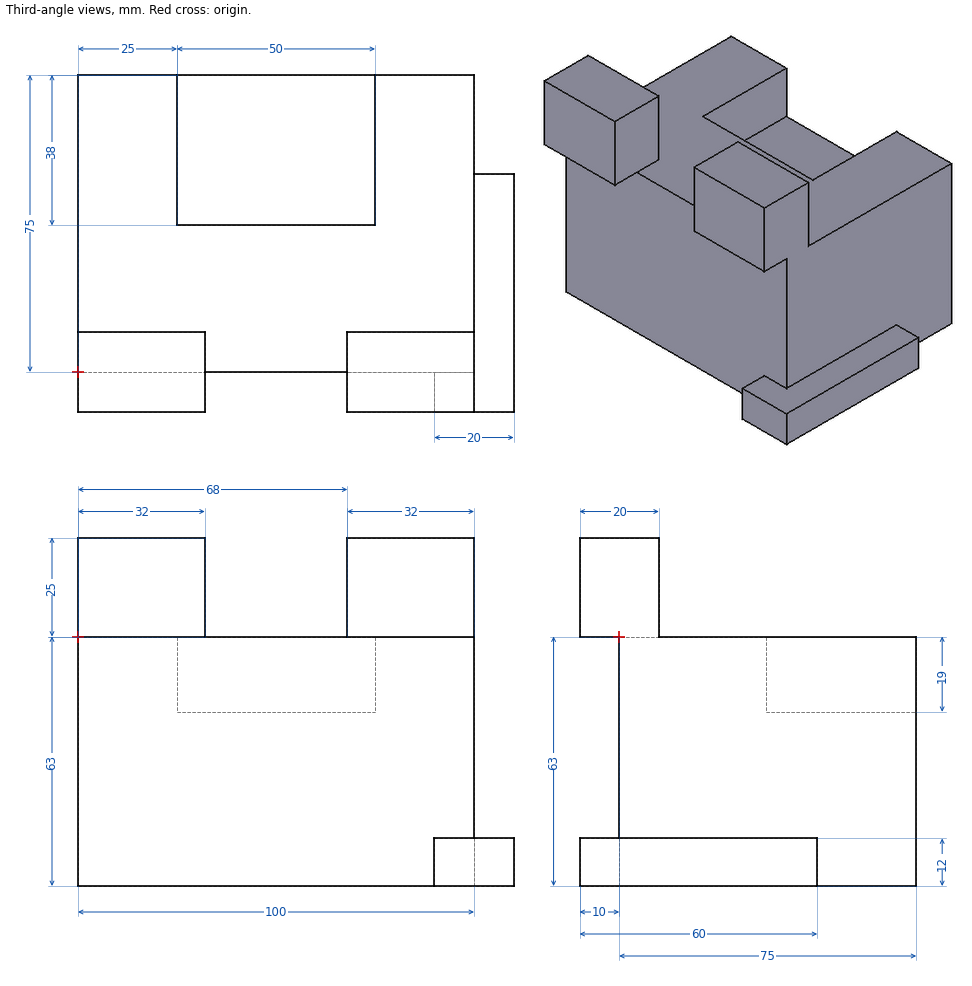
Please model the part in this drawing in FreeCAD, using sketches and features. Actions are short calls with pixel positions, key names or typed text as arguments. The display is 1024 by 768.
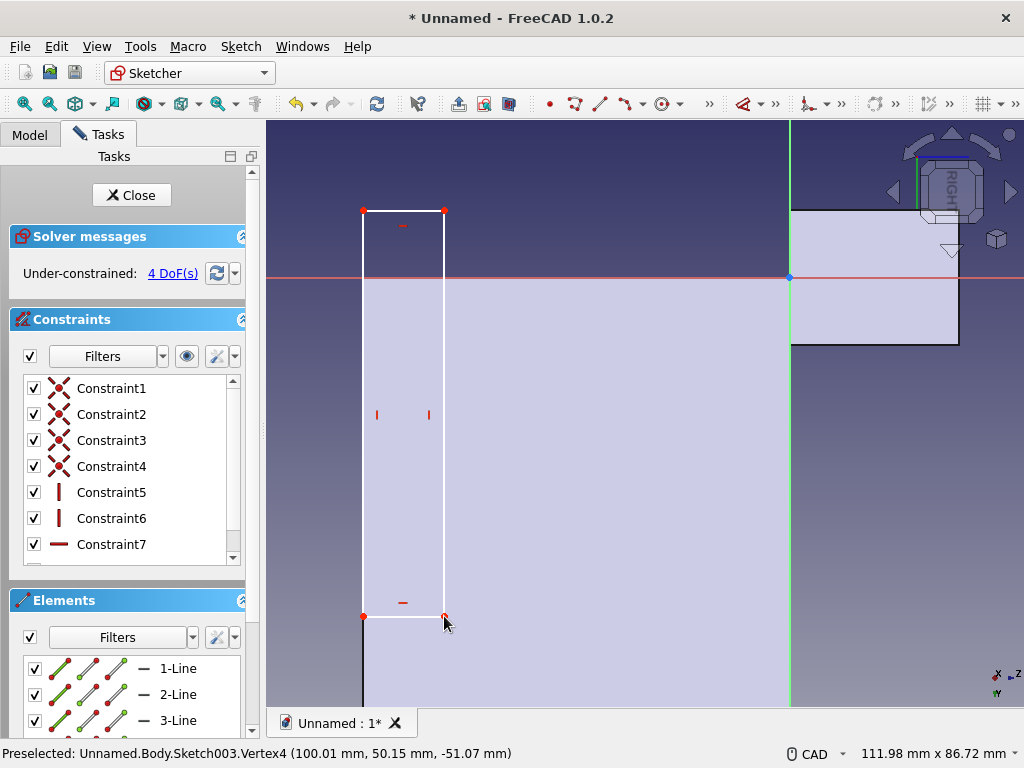
click(742, 104)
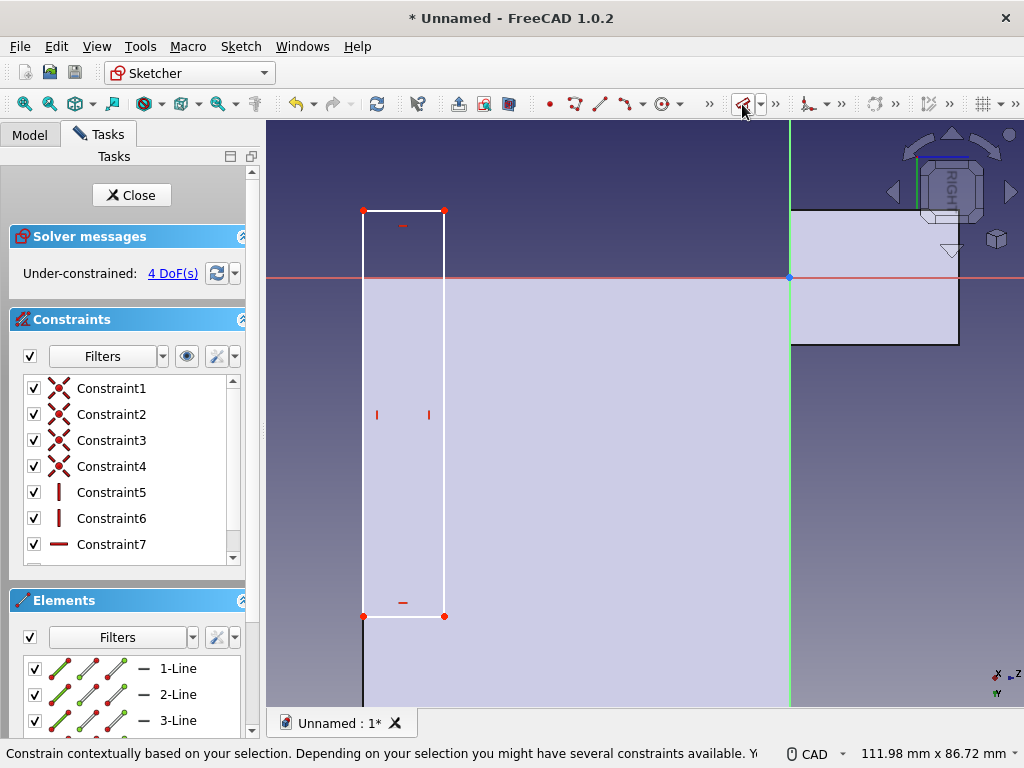
click(363, 333)
click(329, 414)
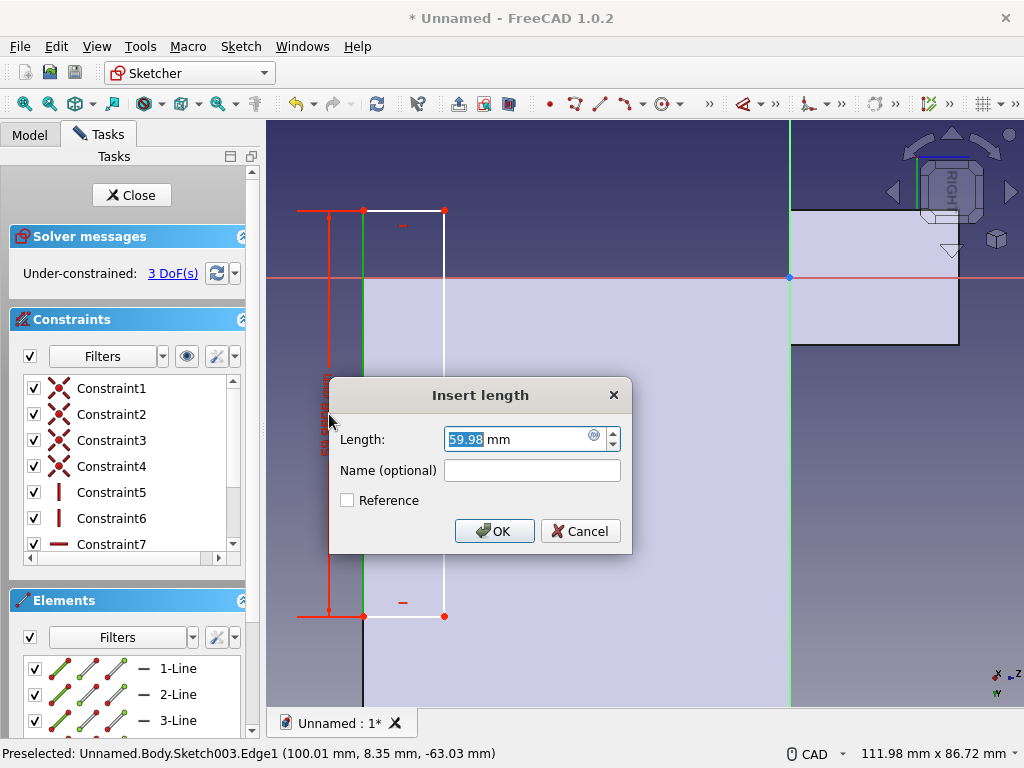
text(60)
key(Return)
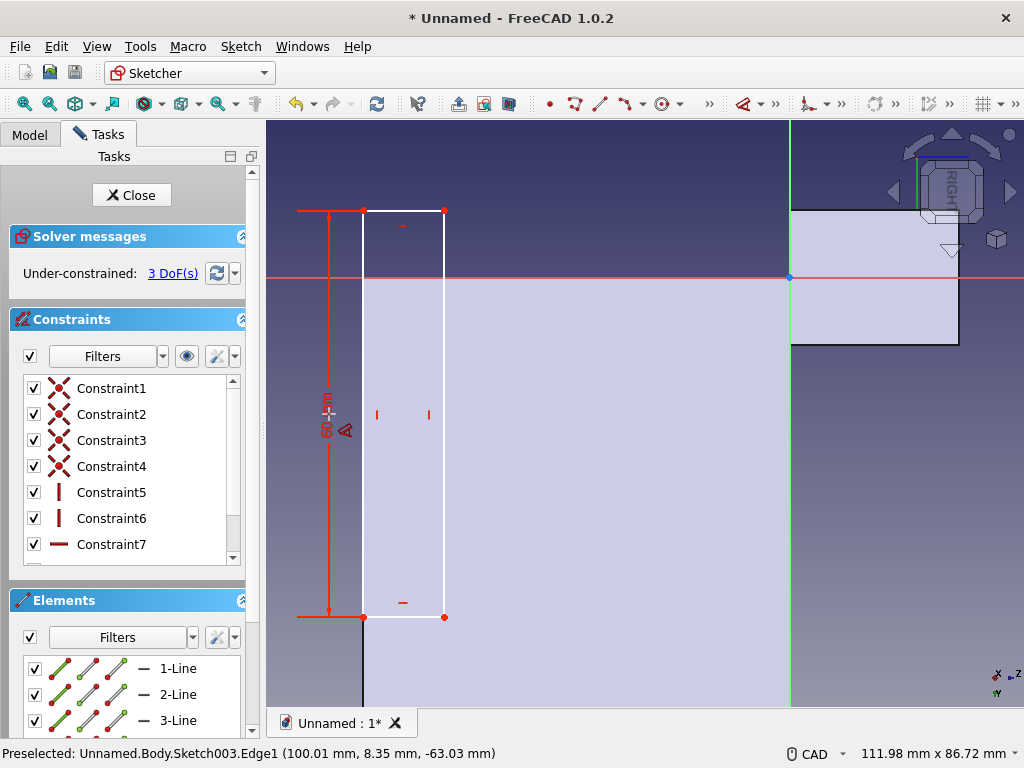
click(387, 617)
click(404, 651)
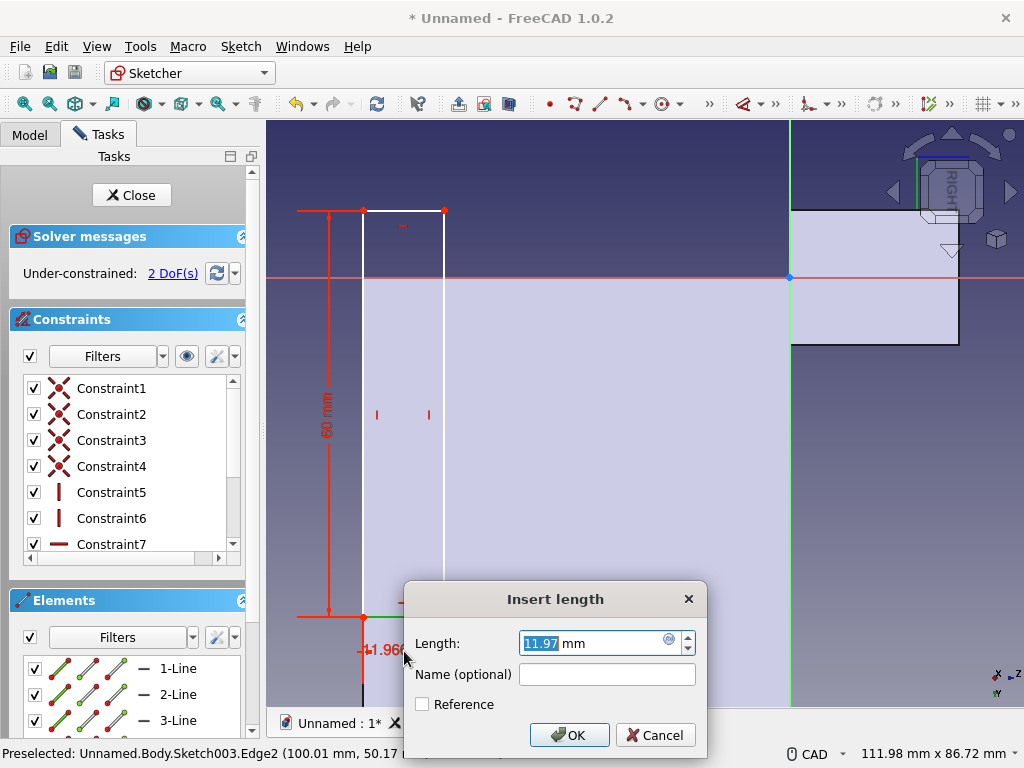
text(12)
key(Return)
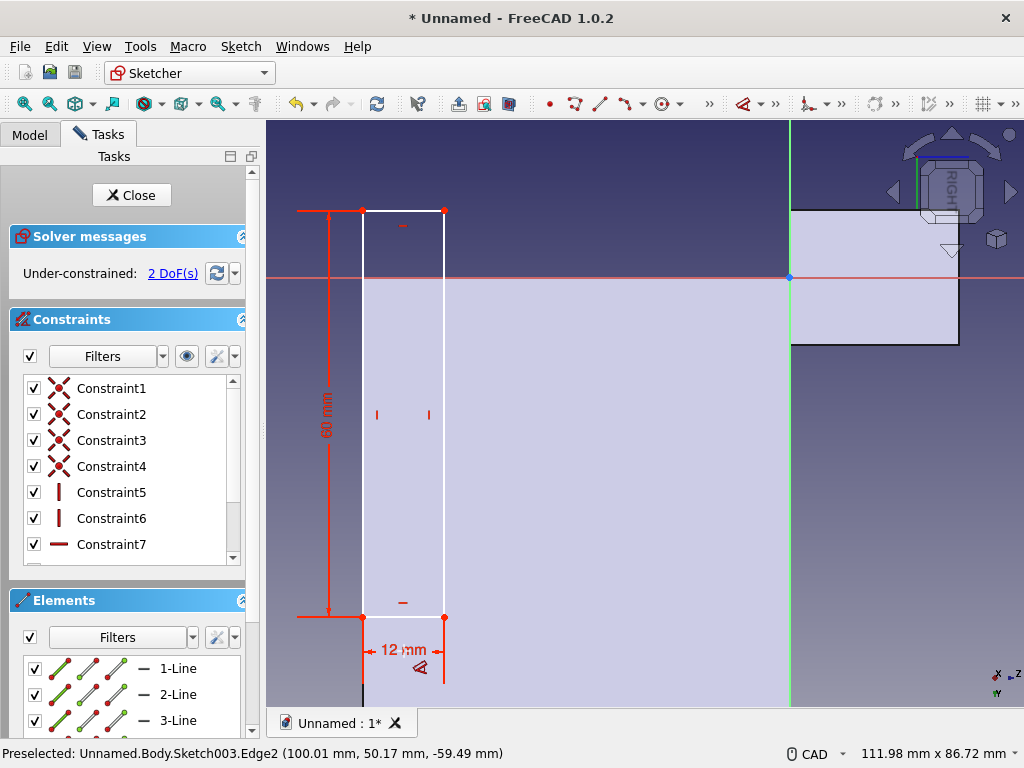
click(363, 211)
click(576, 177)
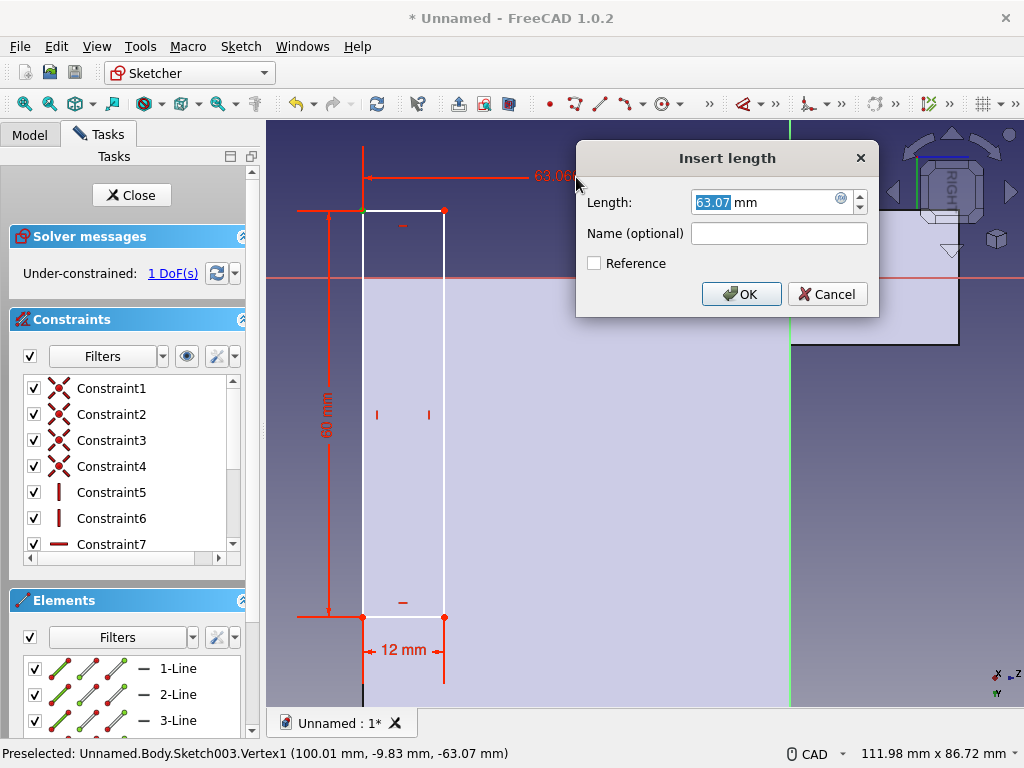
text(63)
key(Return)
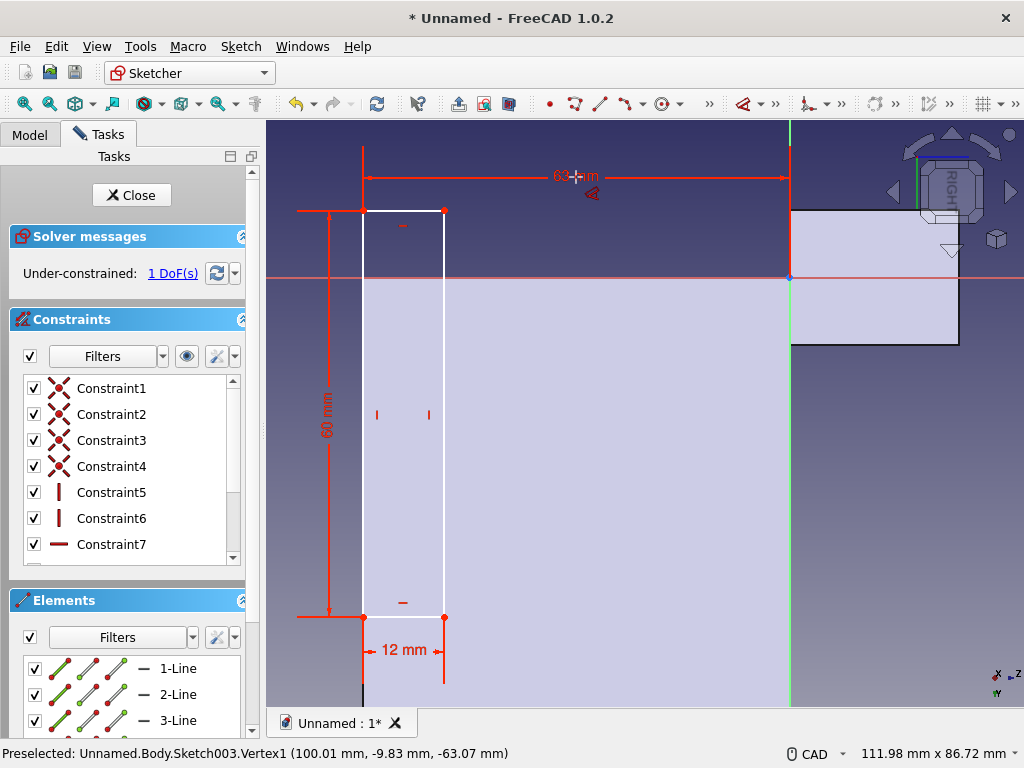
click(363, 211)
click(824, 244)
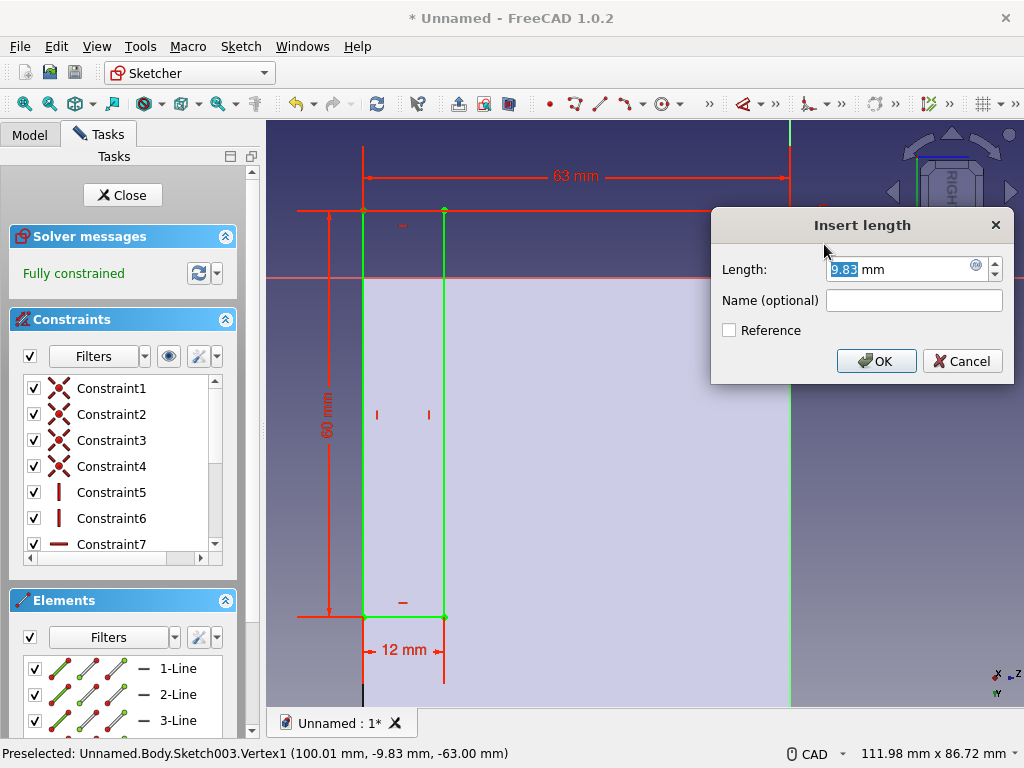
text(10)
key(Return)
key(Escape)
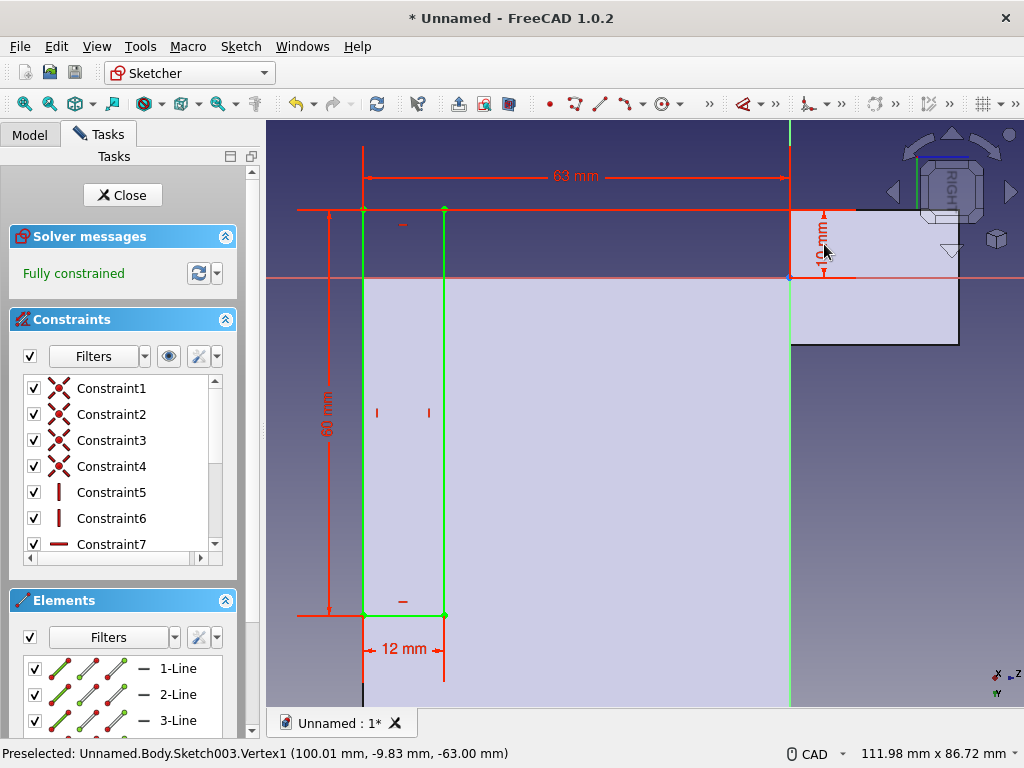
click(123, 195)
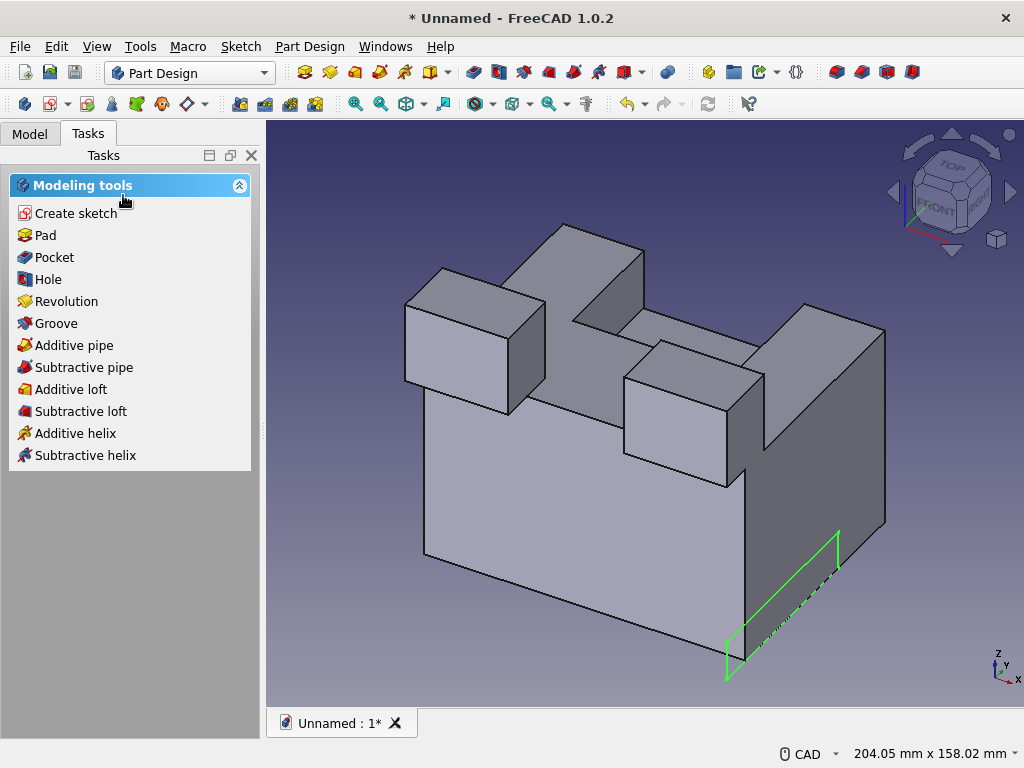
click(305, 72)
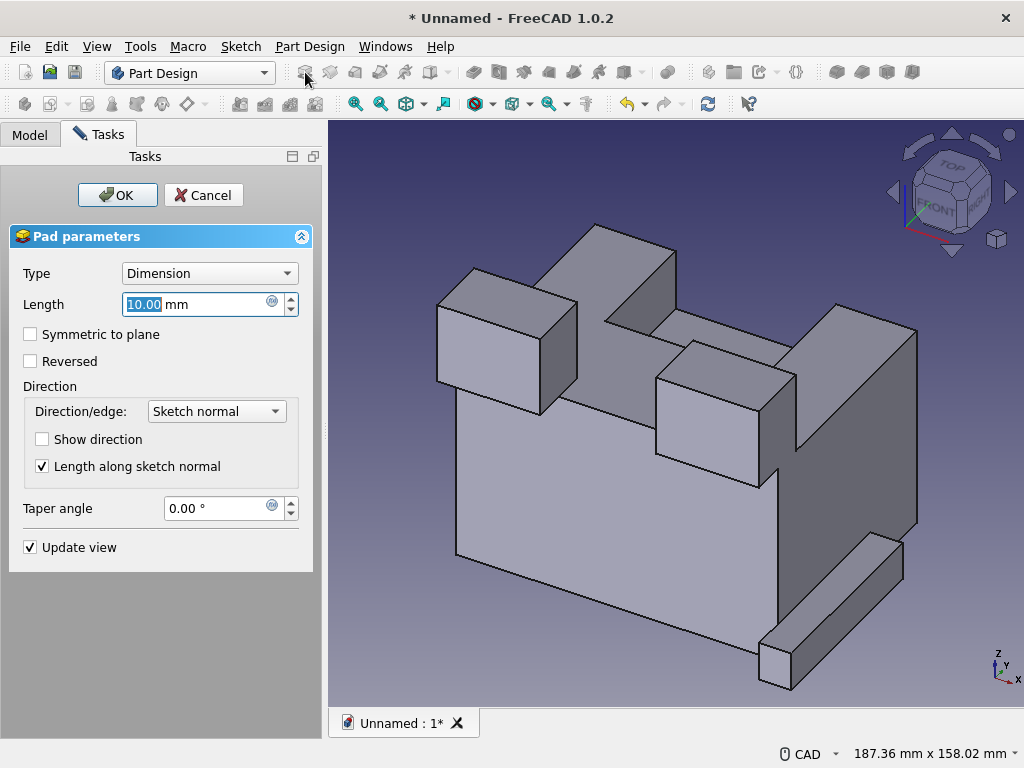
text(20)
key(Tab)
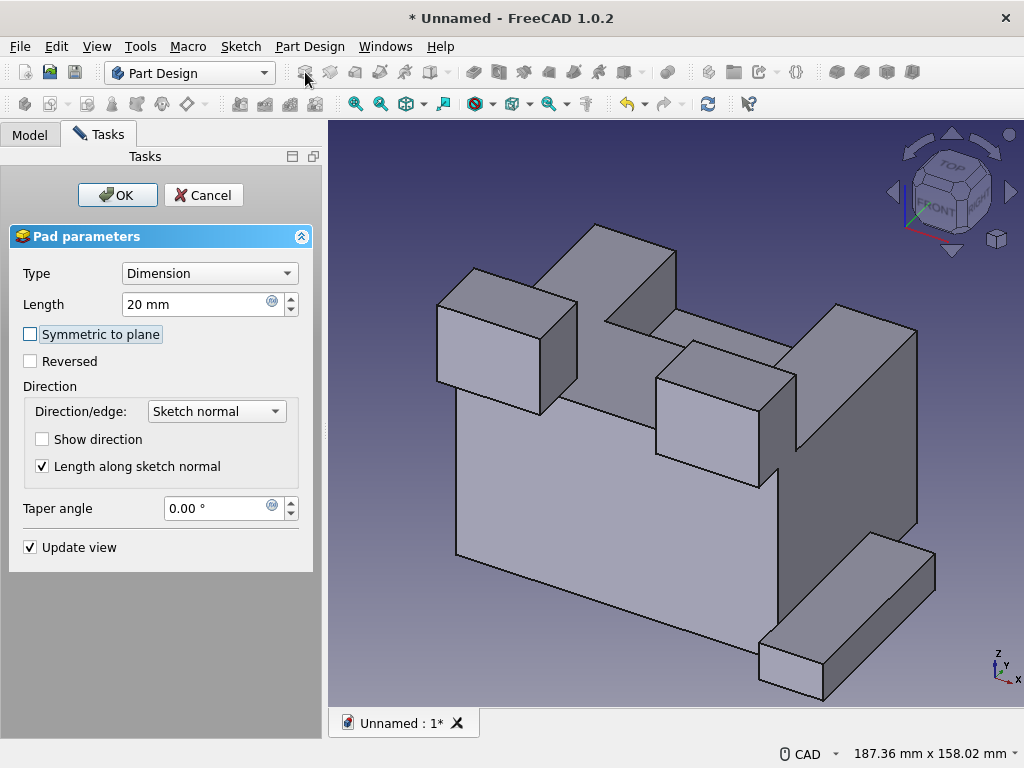
click(31, 334)